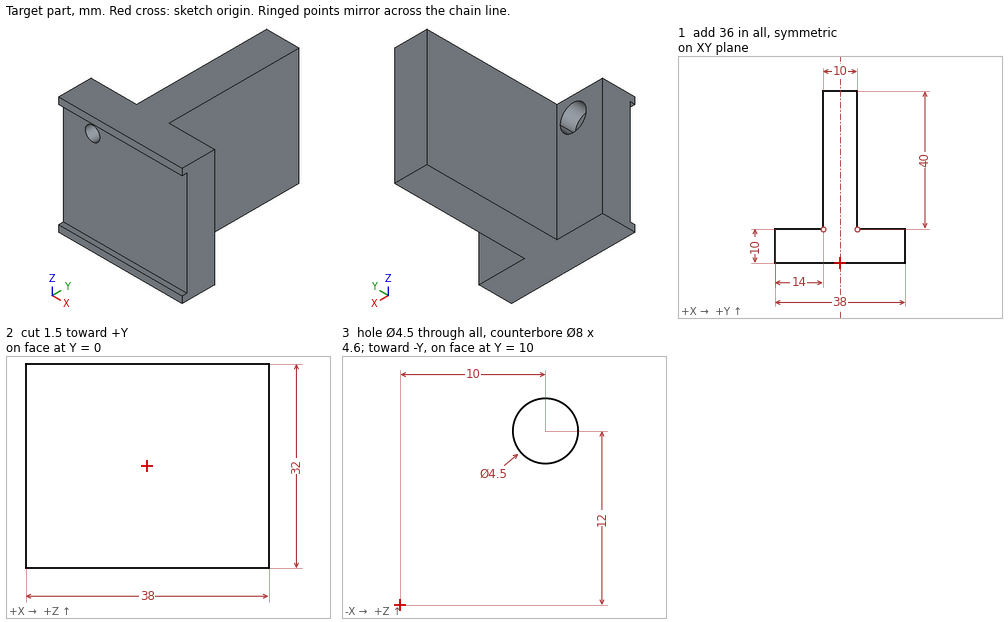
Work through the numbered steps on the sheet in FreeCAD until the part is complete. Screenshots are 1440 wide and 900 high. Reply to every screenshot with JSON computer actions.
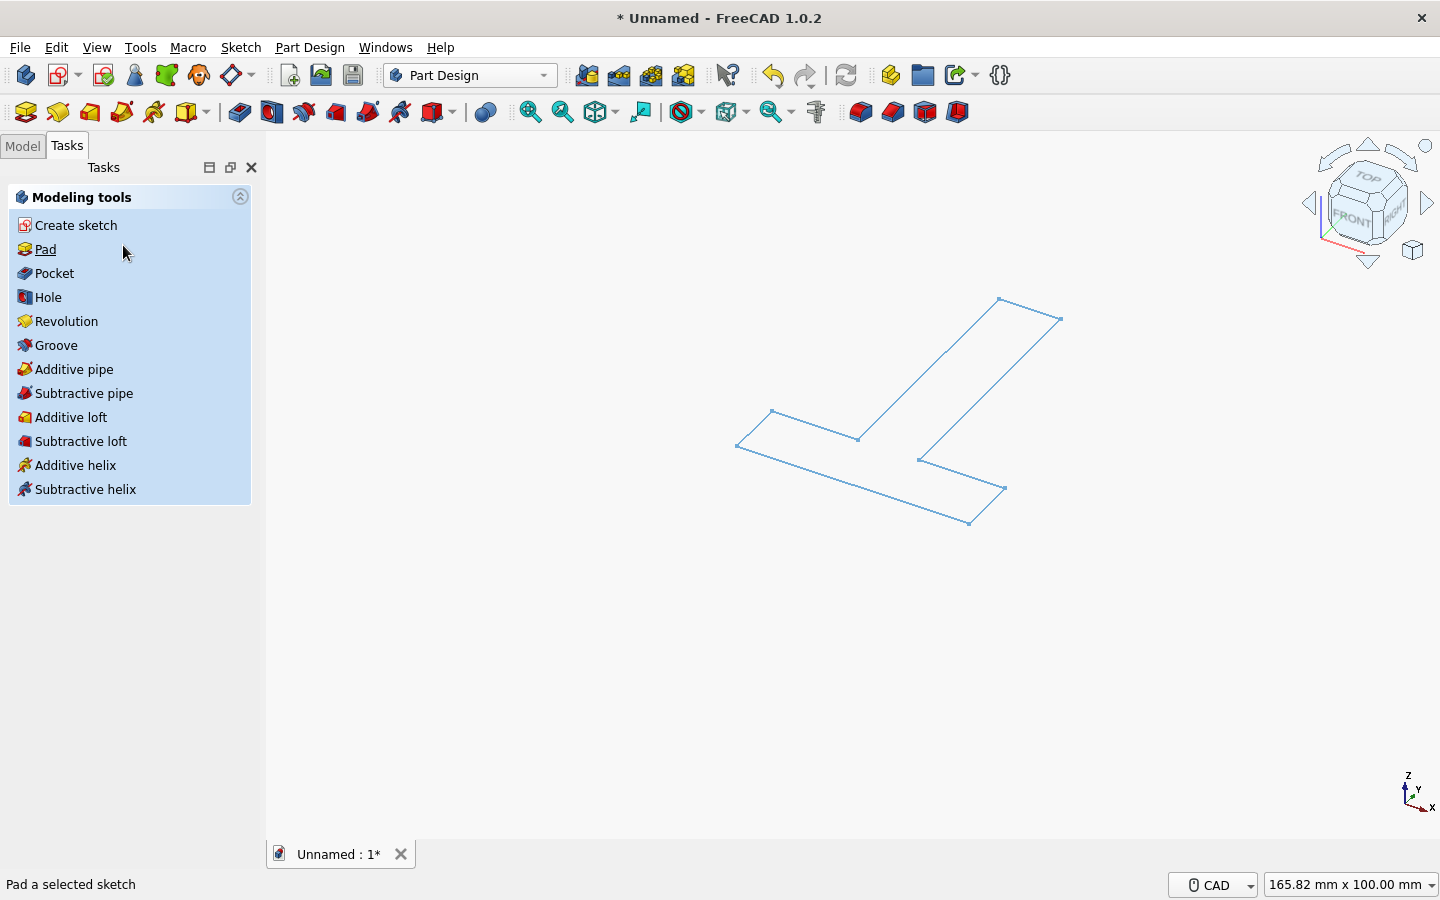
{"action": "left_click", "coordinate": [26, 112]}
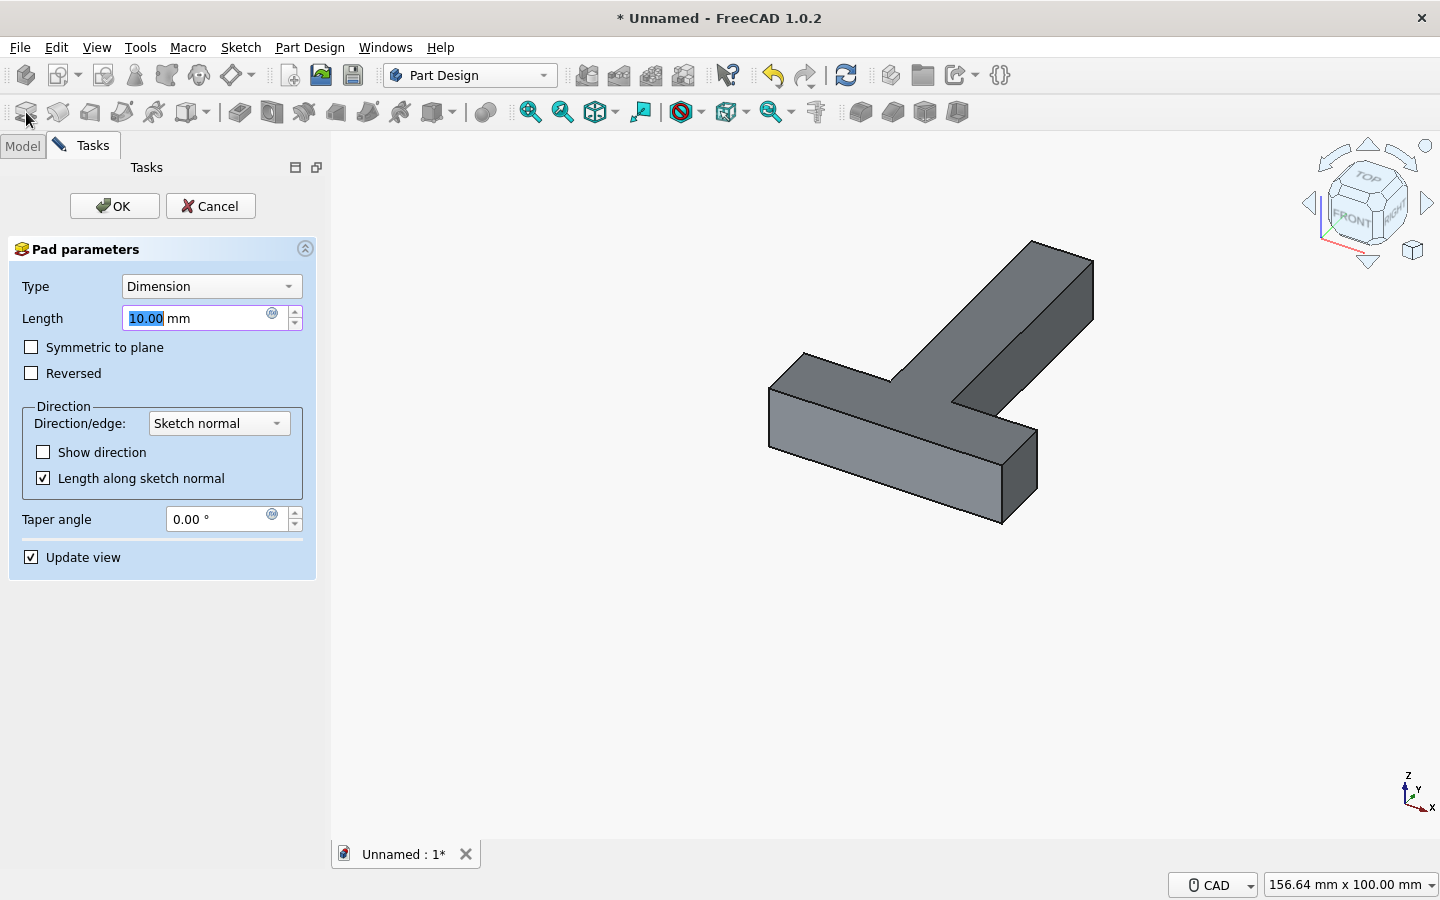
{"action": "type", "text": "36"}
{"action": "key", "text": "Tab"}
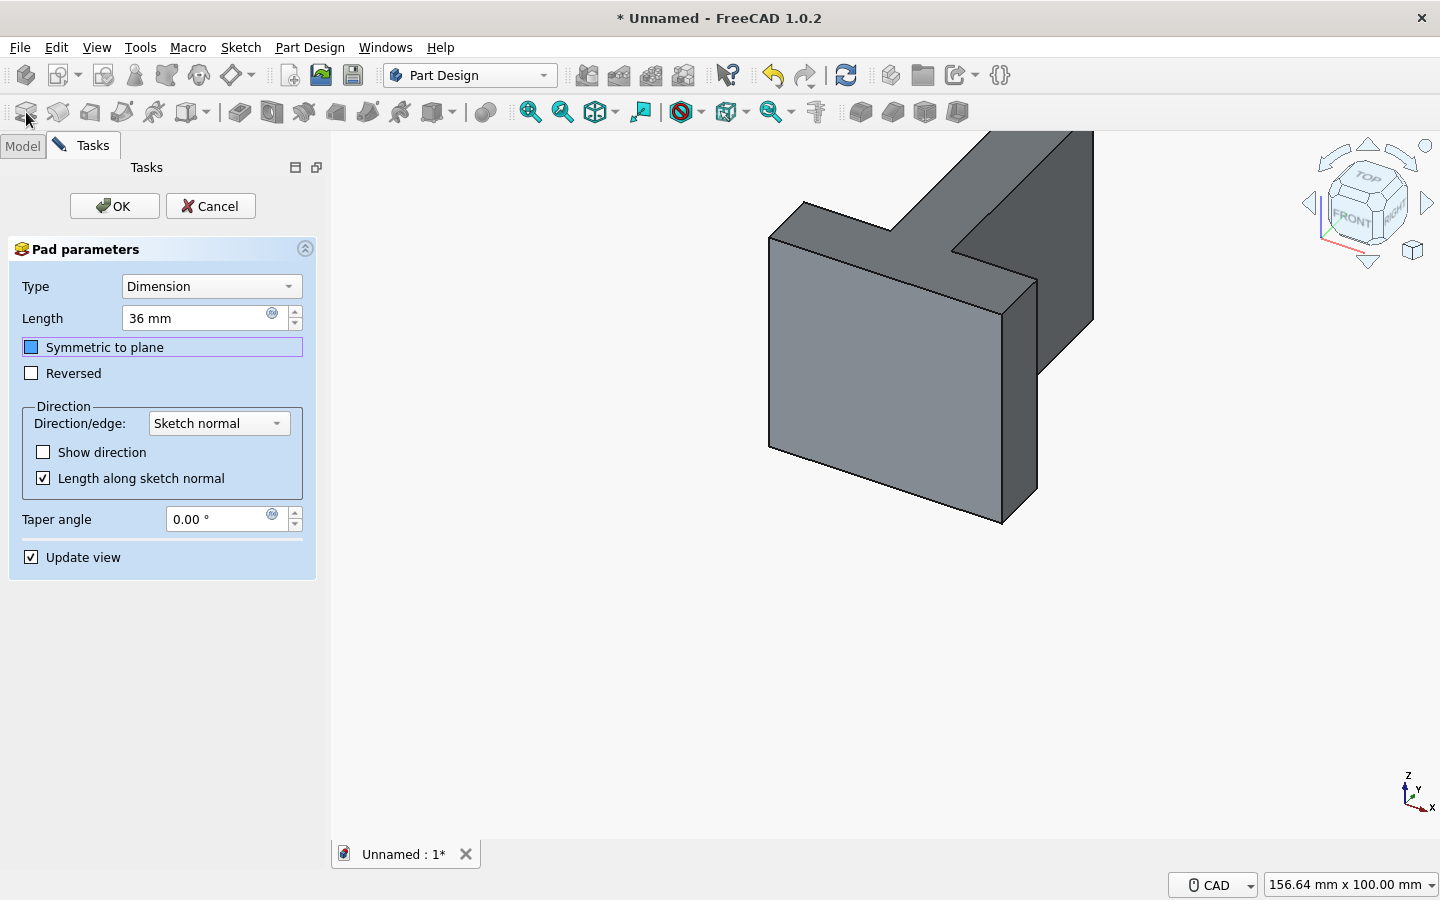
{"action": "left_click", "coordinate": [30, 347]}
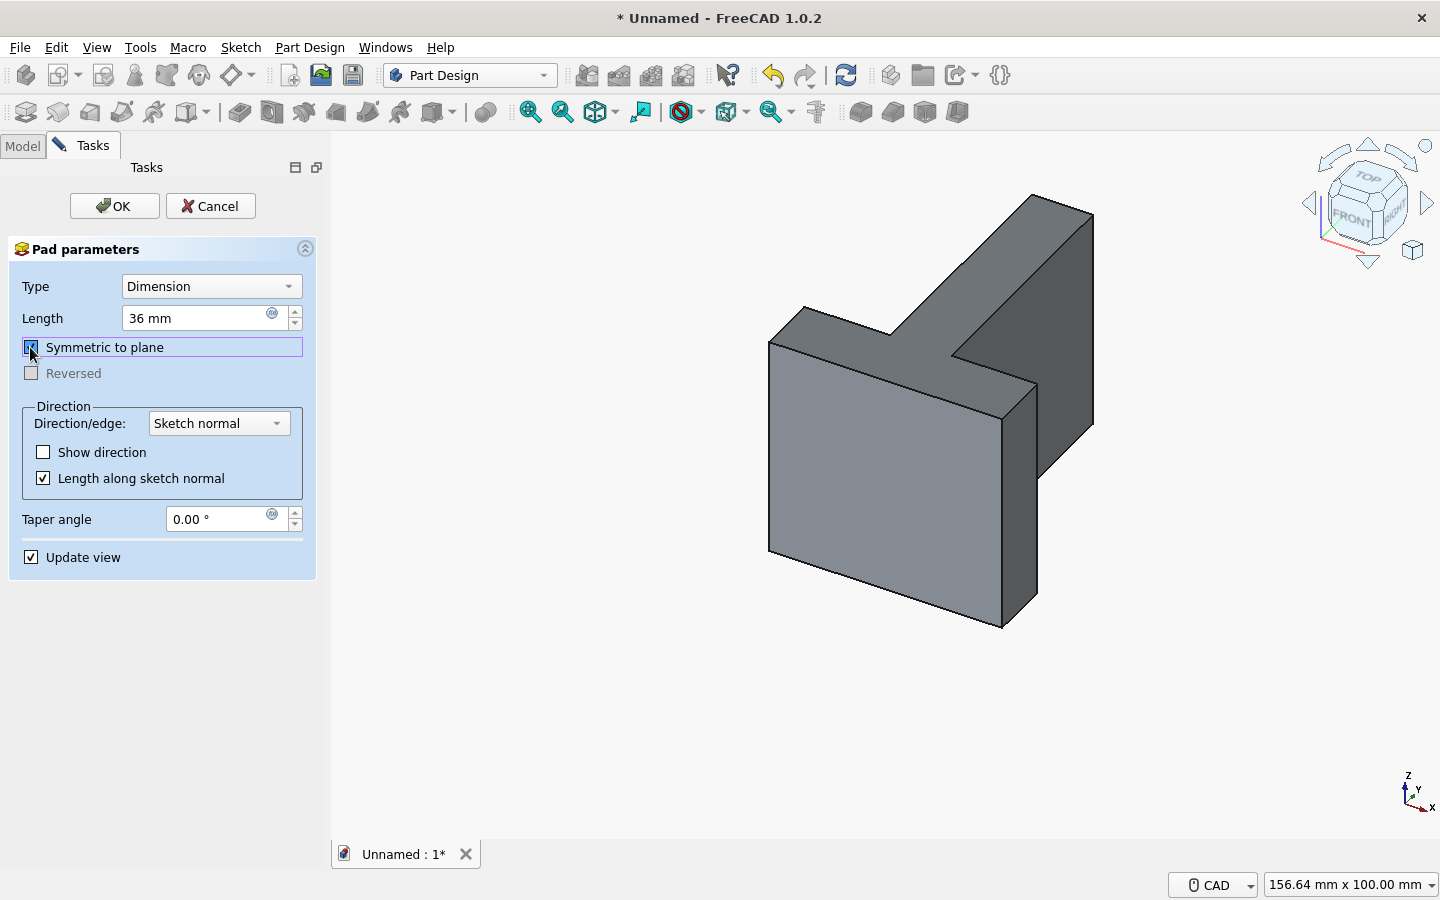
{"action": "left_click", "coordinate": [115, 206]}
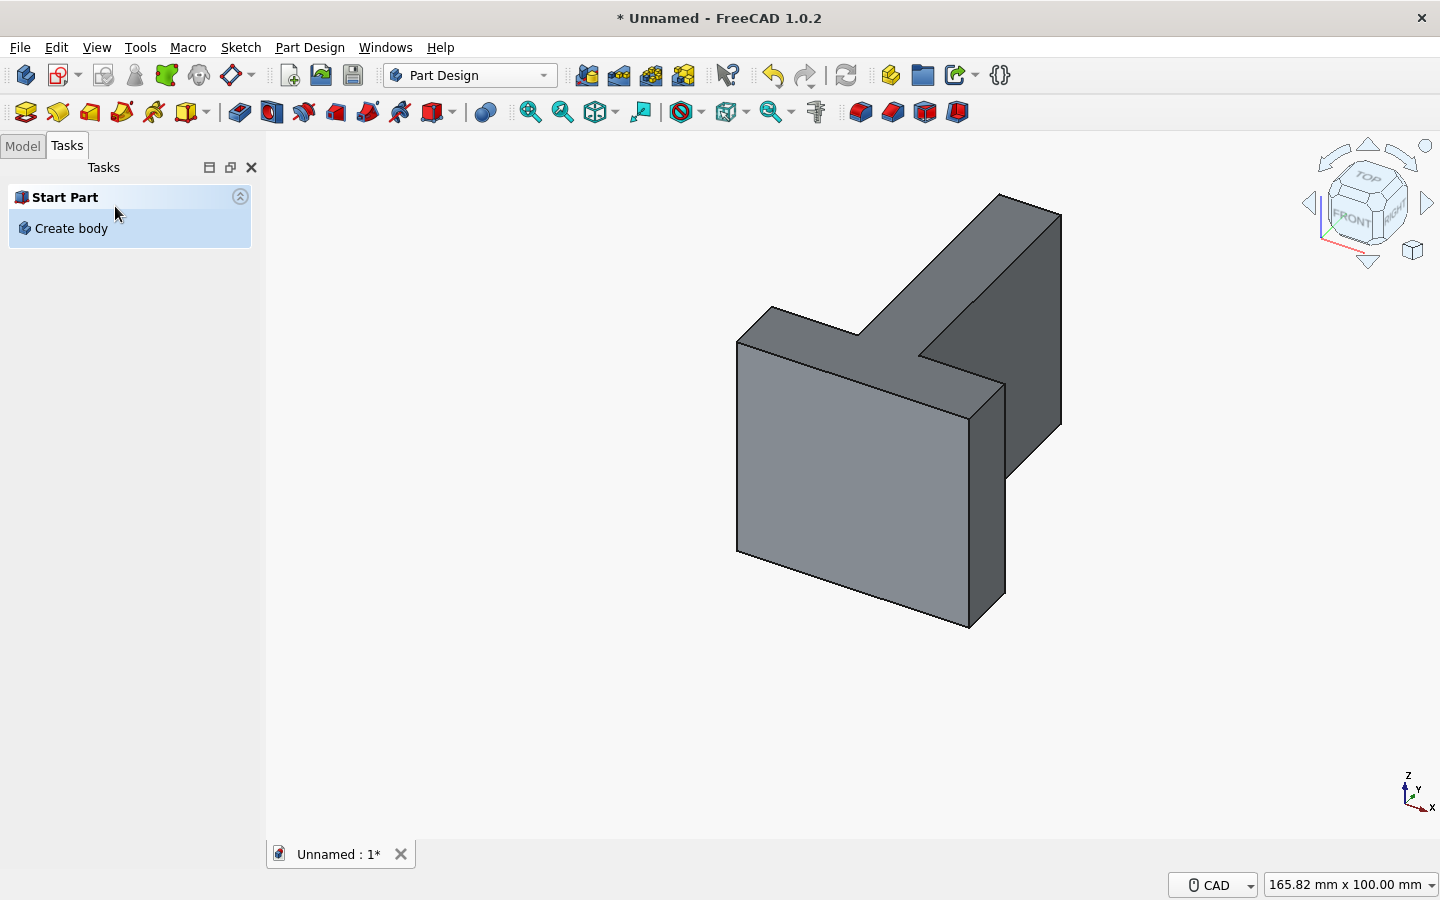
{"action": "left_click", "coordinate": [853, 484]}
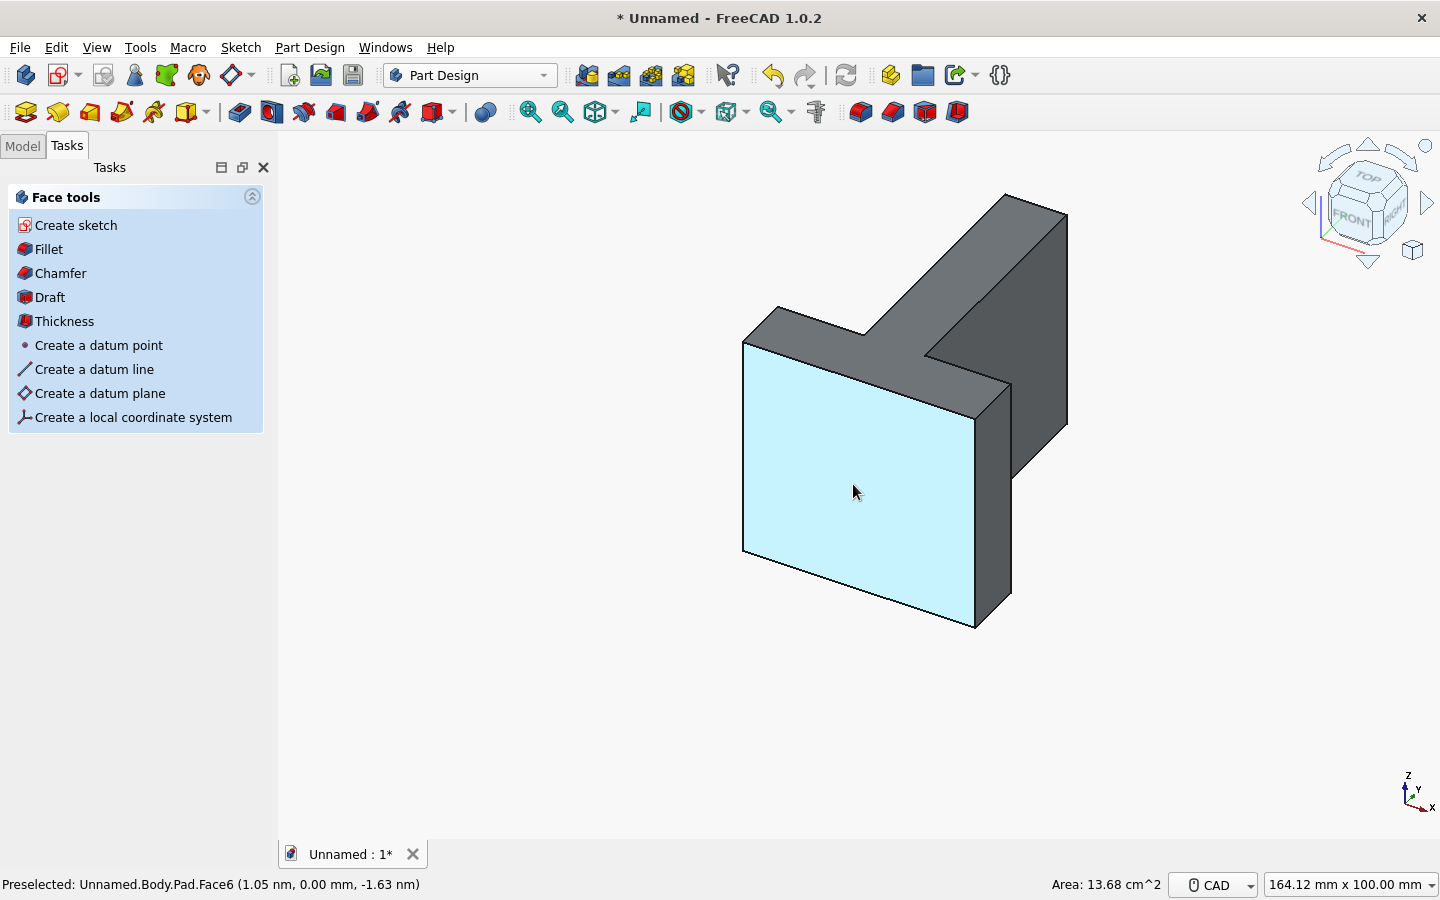
{"action": "left_click", "coordinate": [58, 76]}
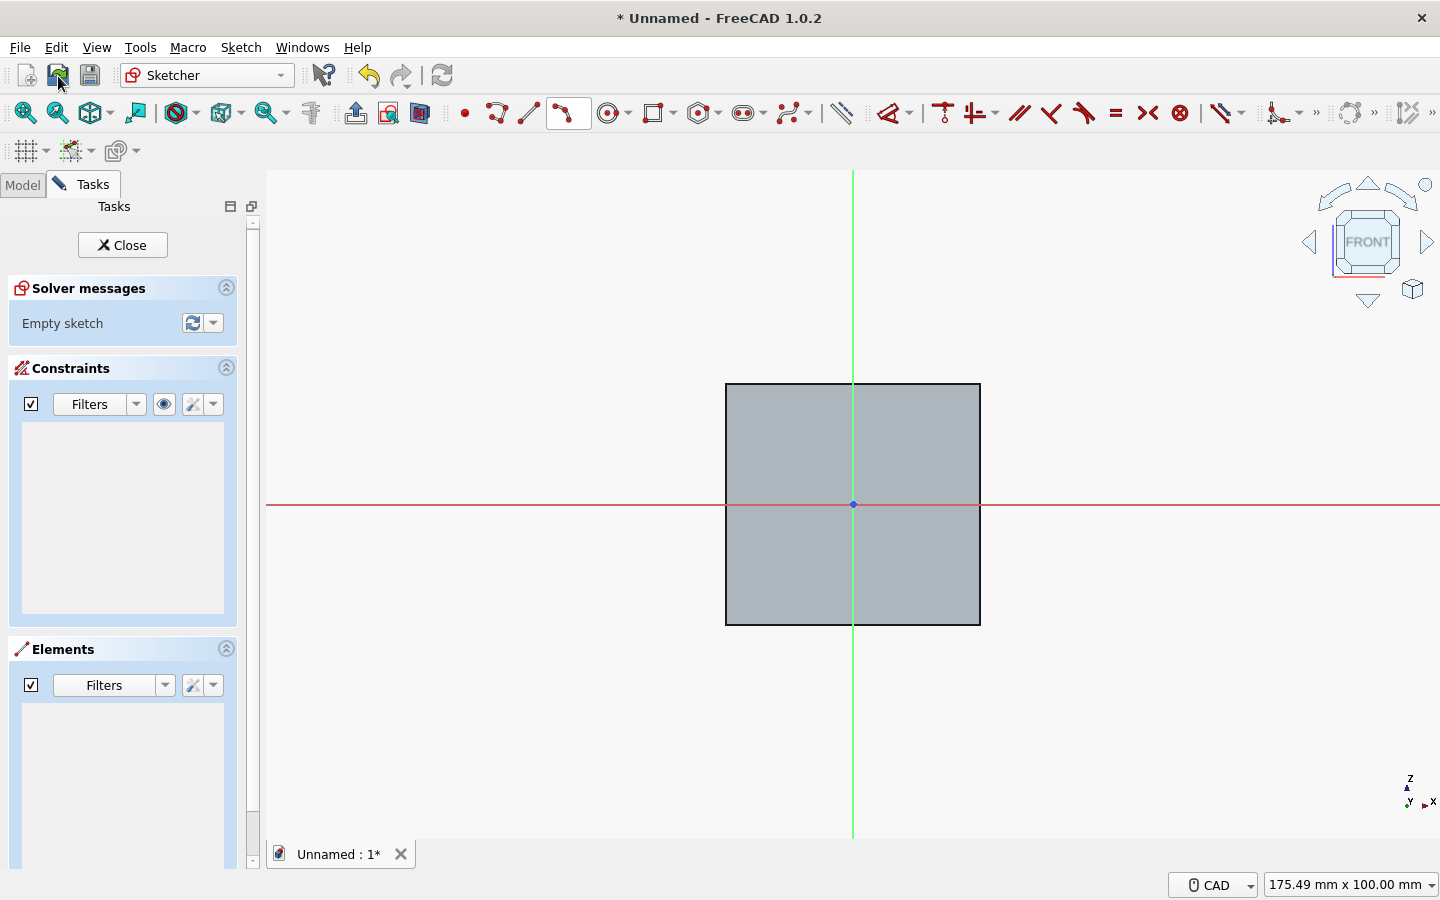
{"action": "scroll", "coordinate": [909, 504], "scroll_direction": "up", "scroll_amount": 4}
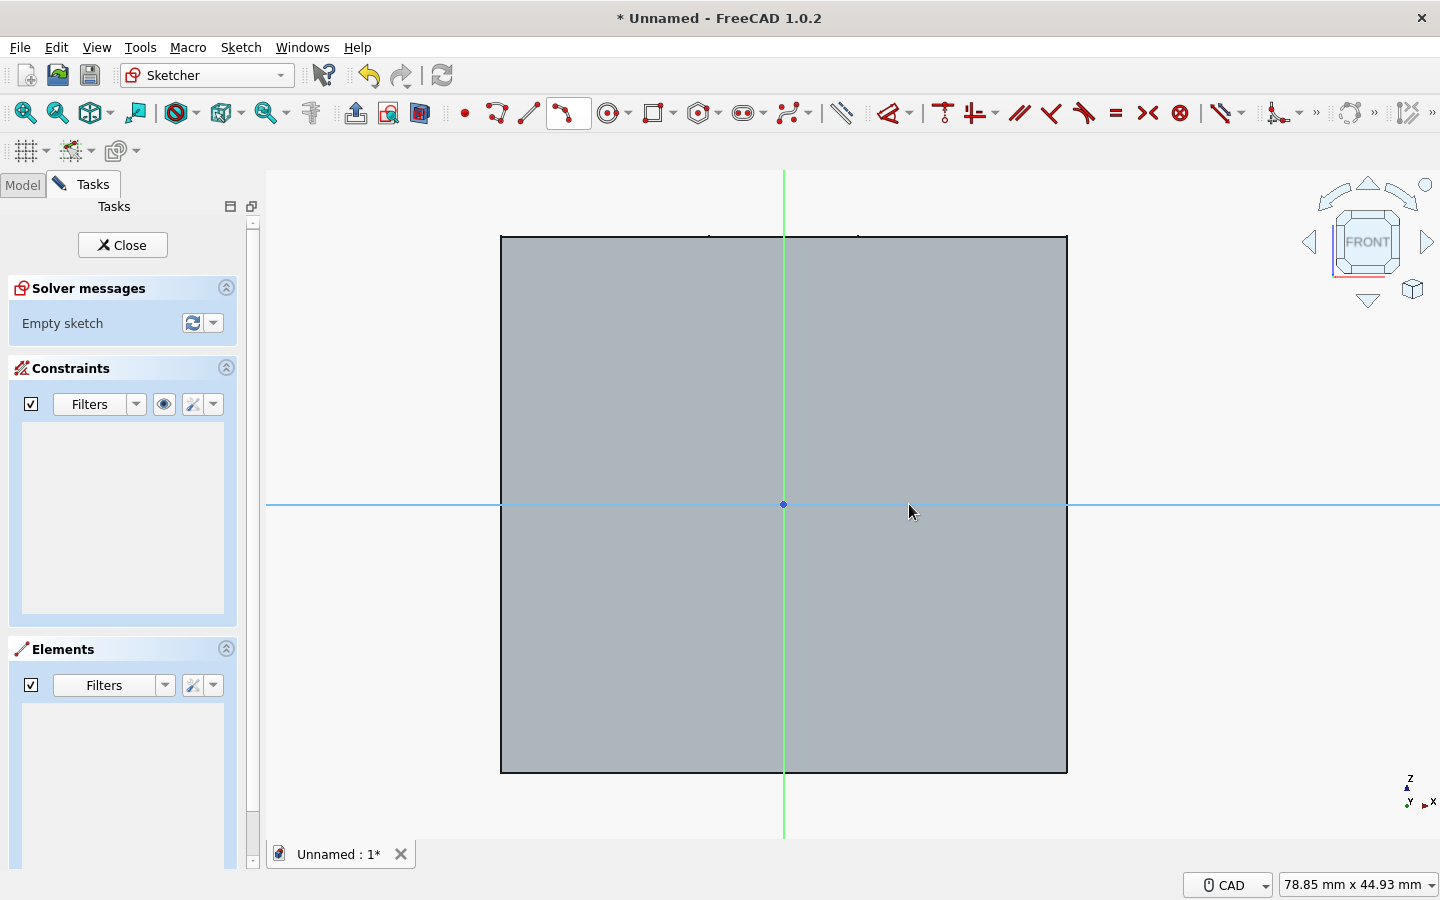
{"action": "left_click", "coordinate": [676, 114]}